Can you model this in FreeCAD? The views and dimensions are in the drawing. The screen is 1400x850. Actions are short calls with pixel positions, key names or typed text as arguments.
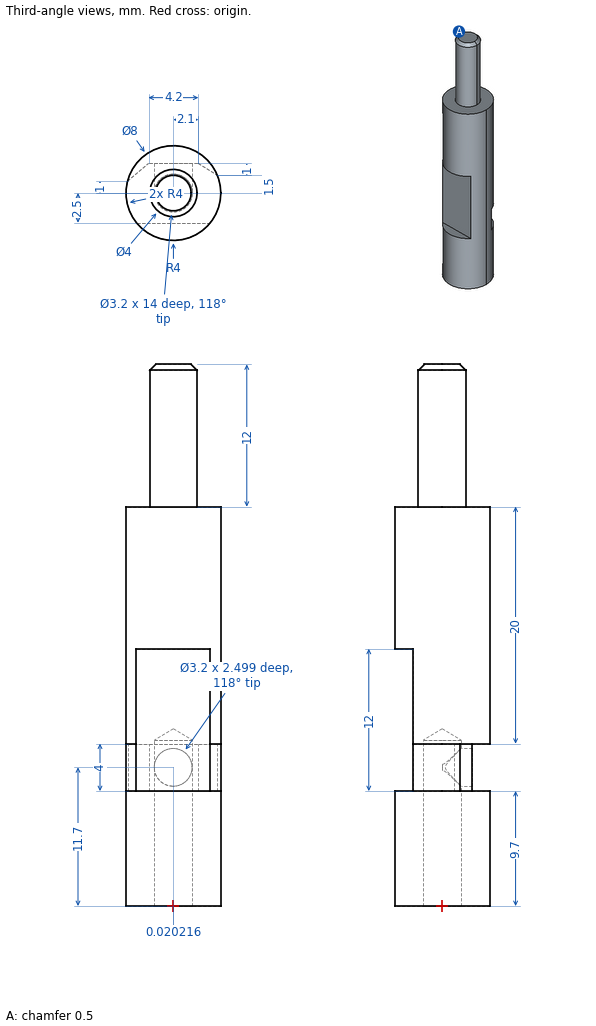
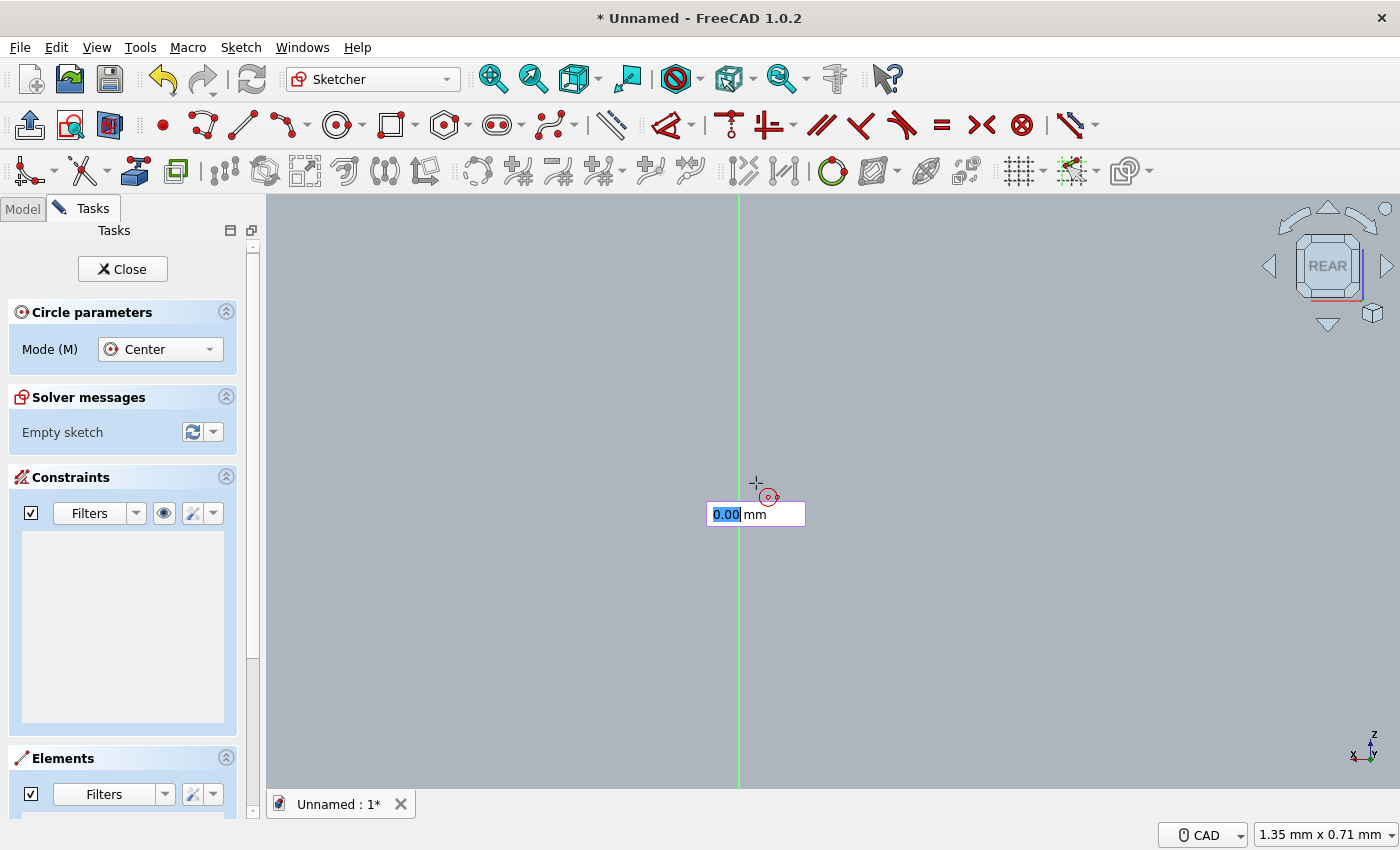
scroll(766, 493, down, 10)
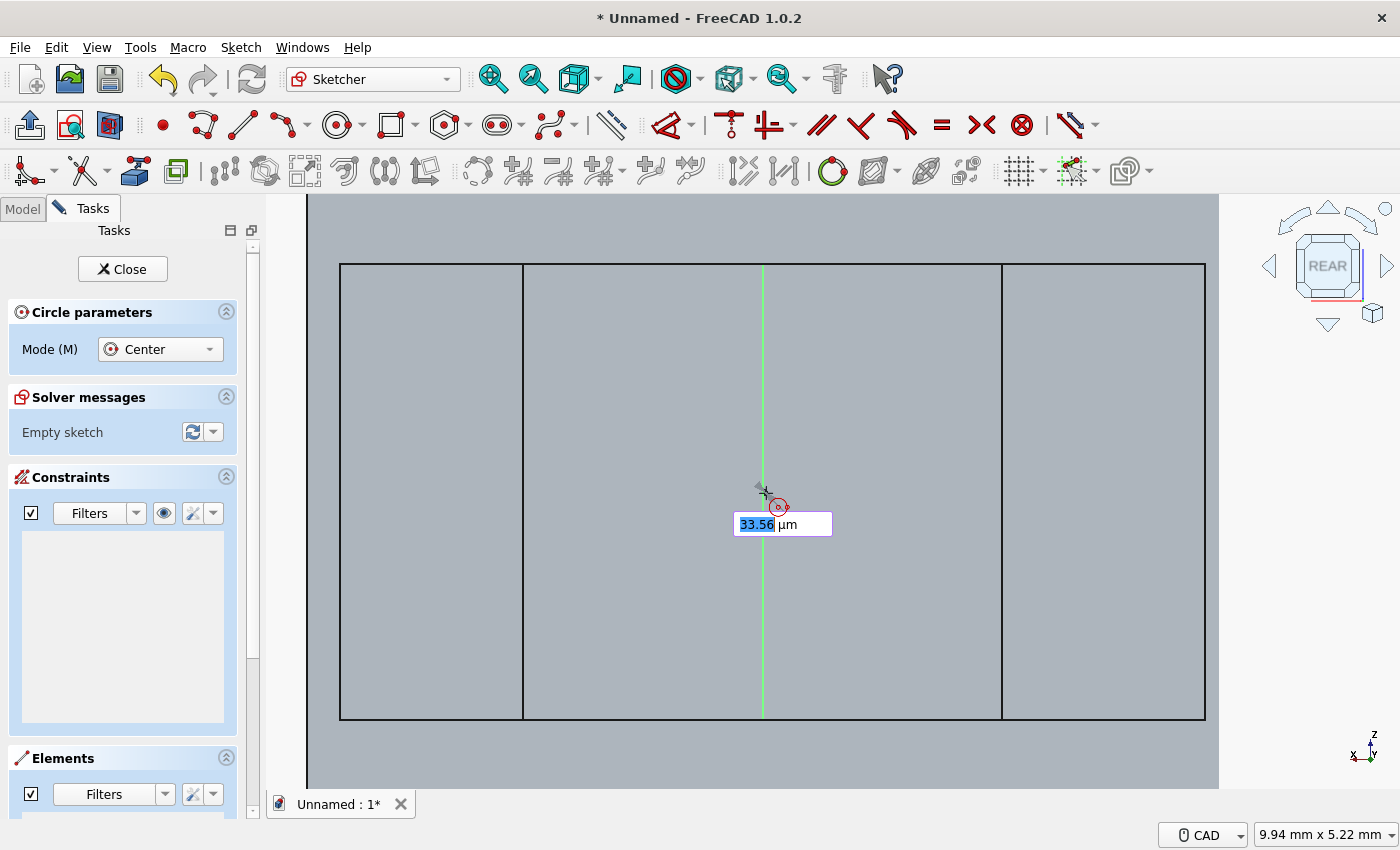
click(894, 363)
key(Escape)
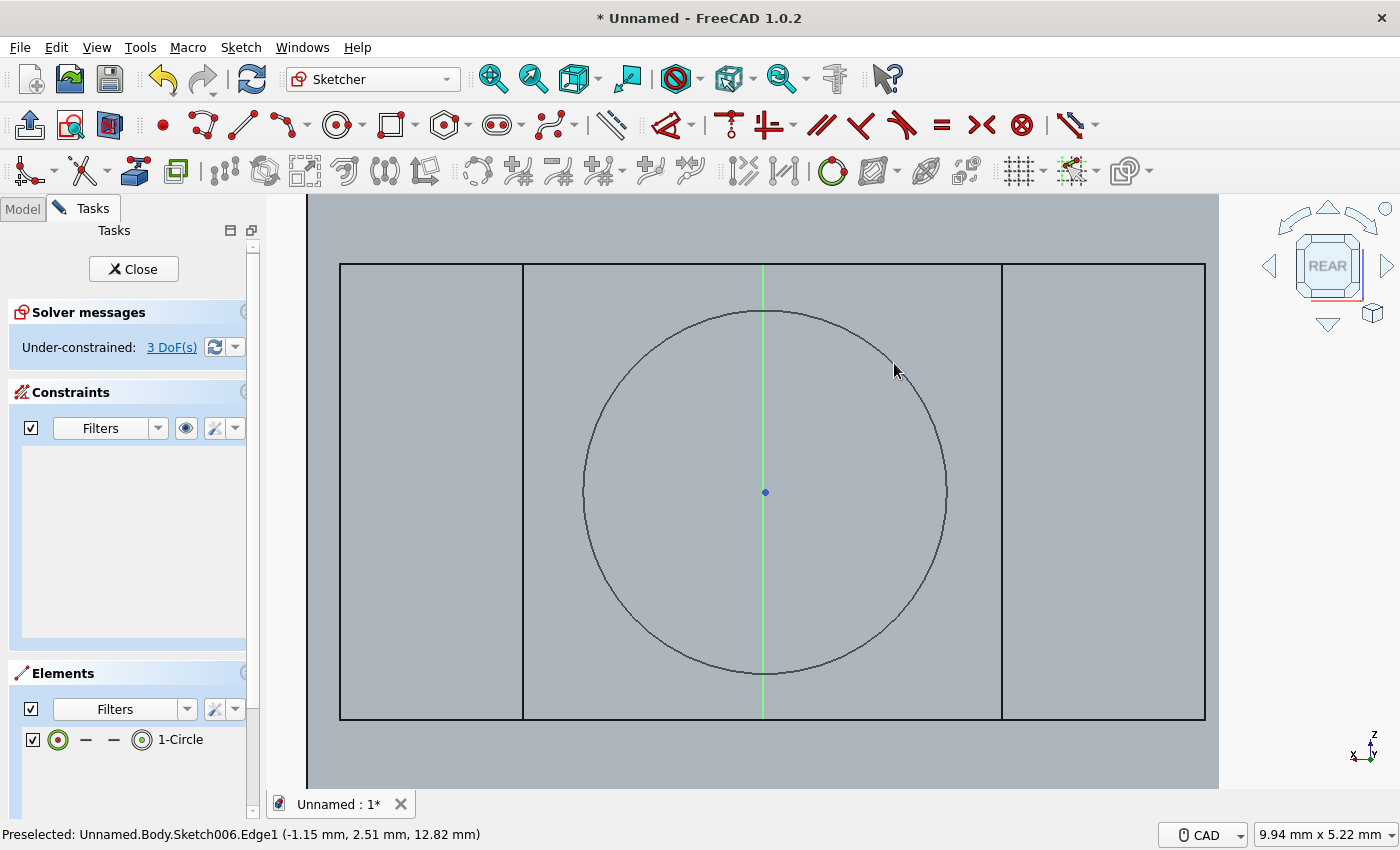
key(d)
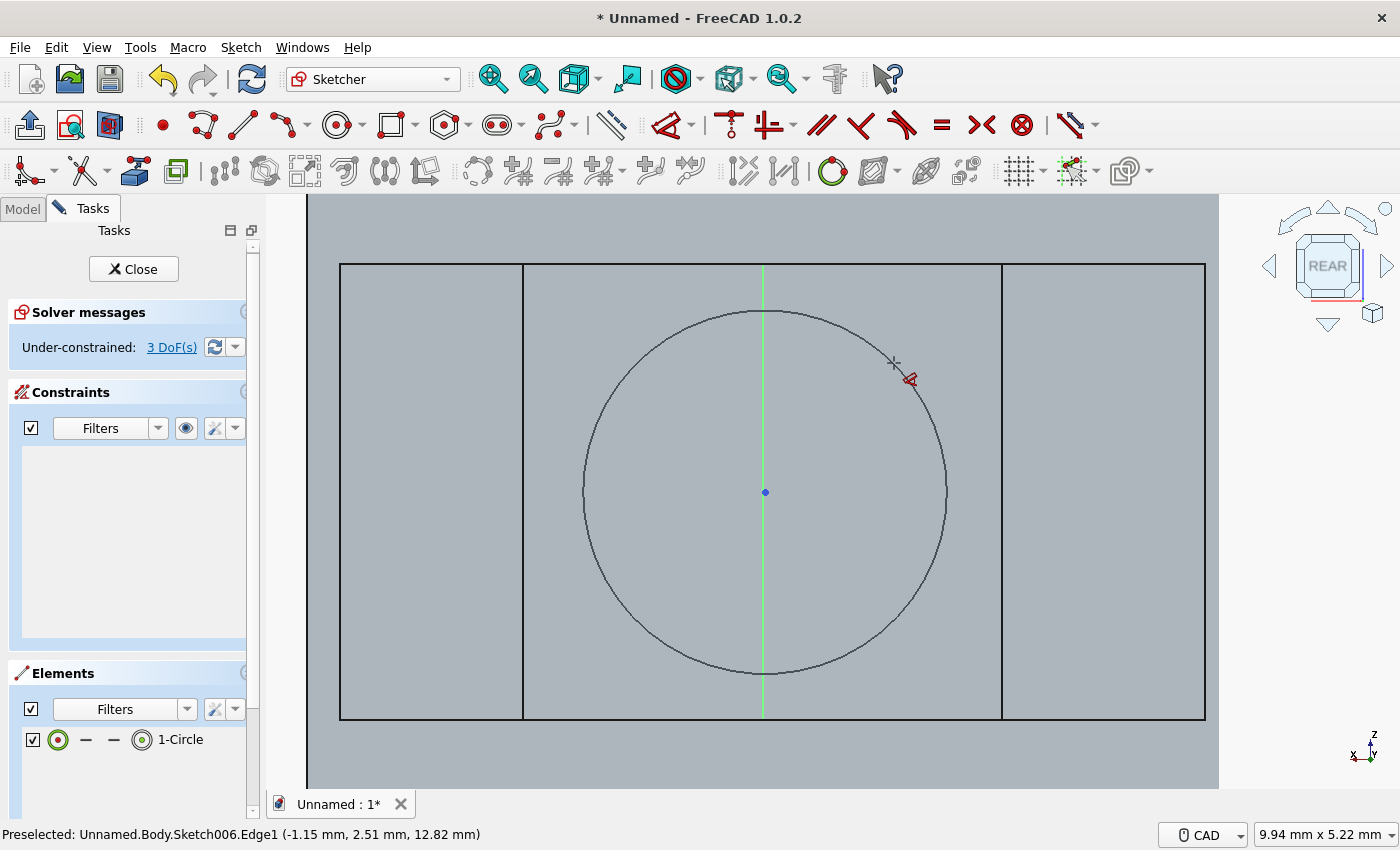
click(893, 363)
click(916, 340)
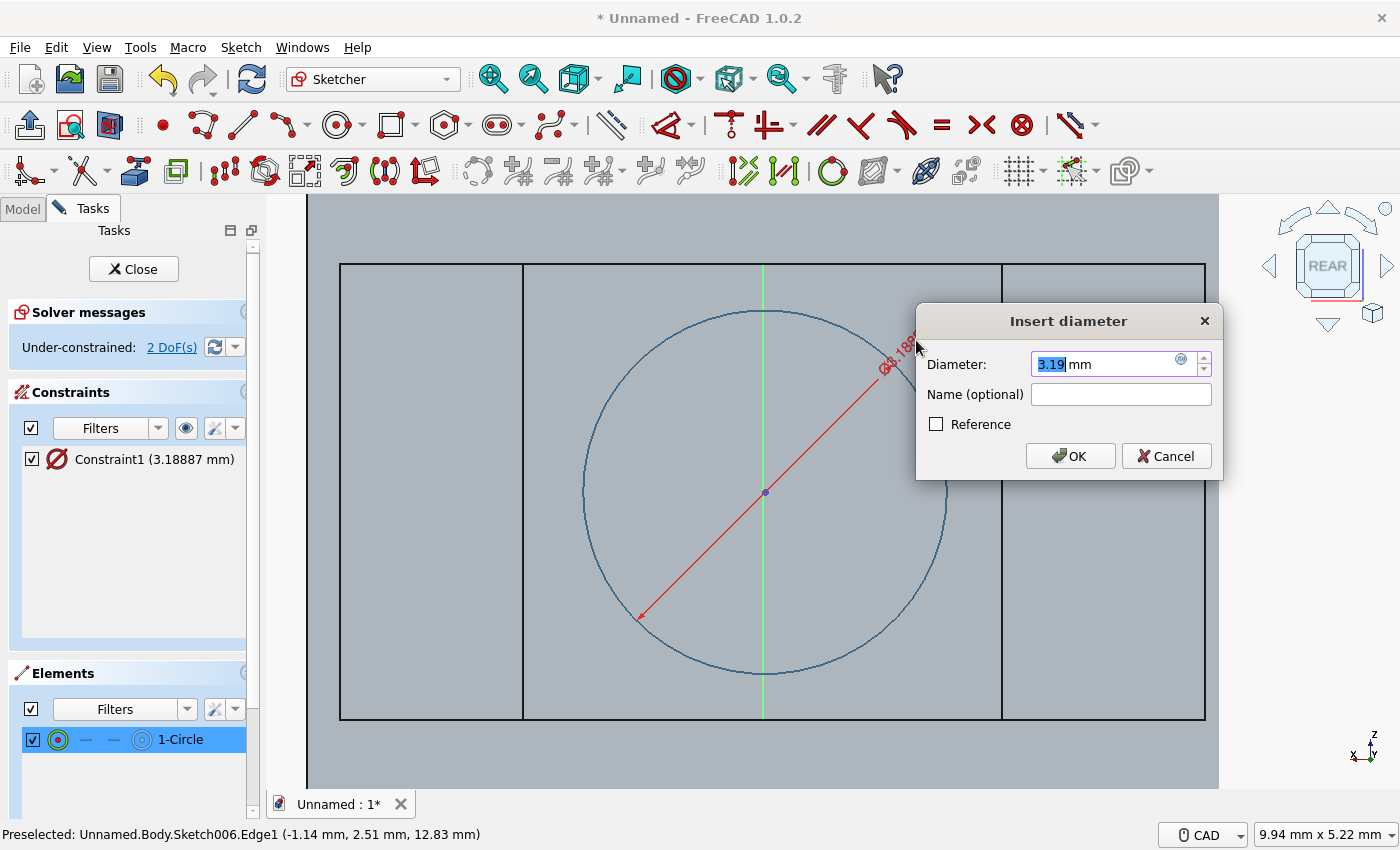
text(3.2)
key(Return)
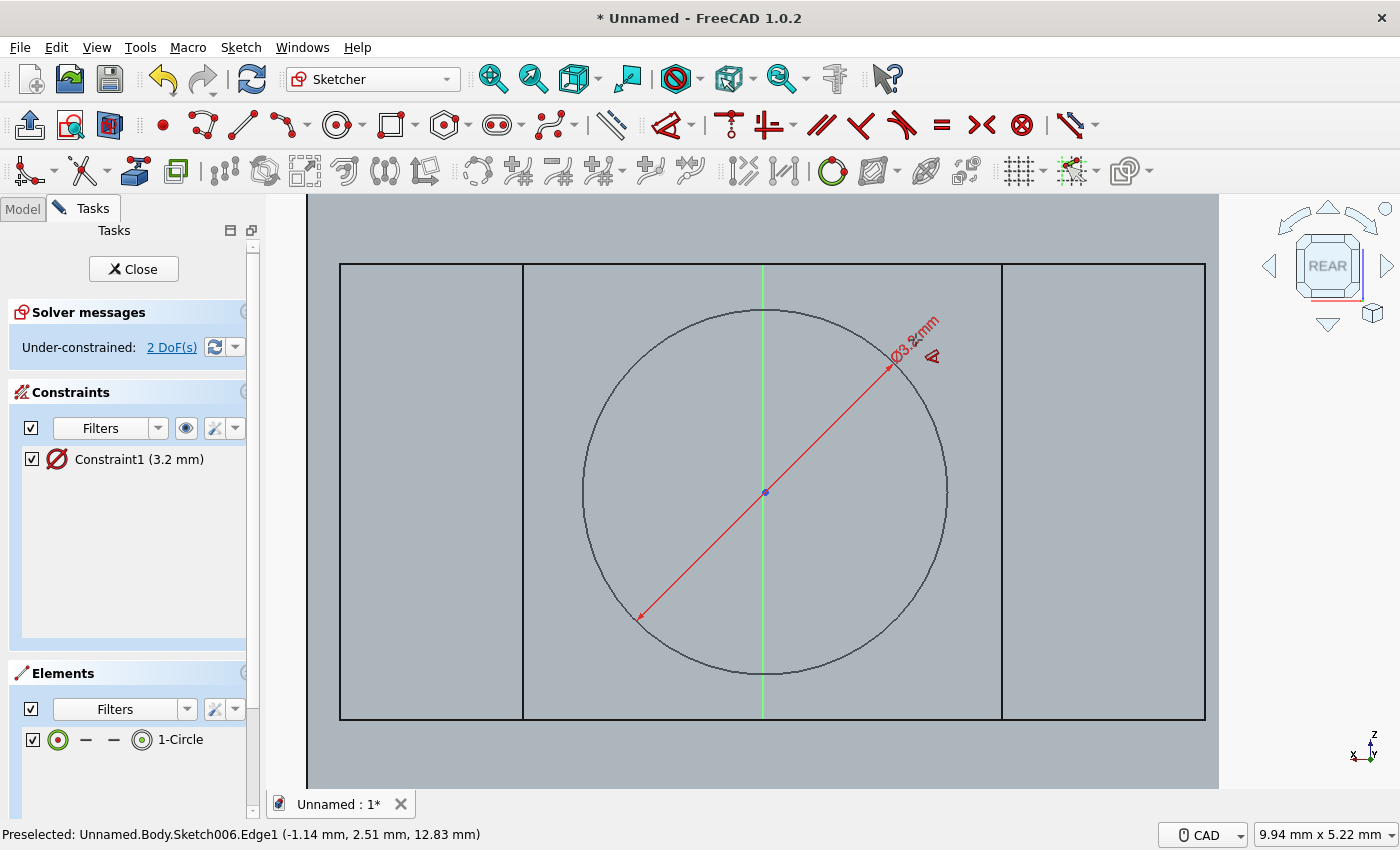
click(765, 492)
click(729, 627)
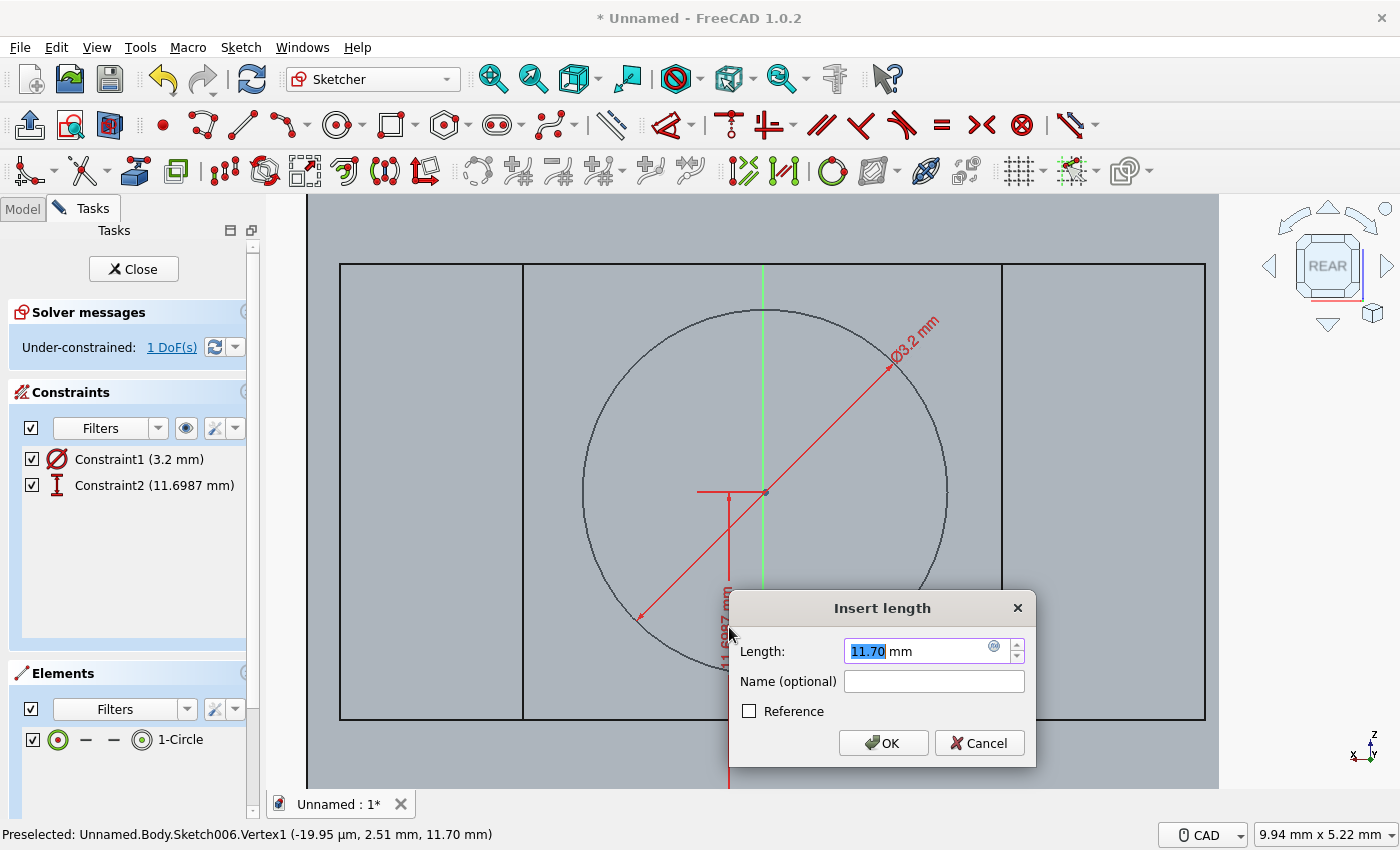
text(11.7)
key(Return)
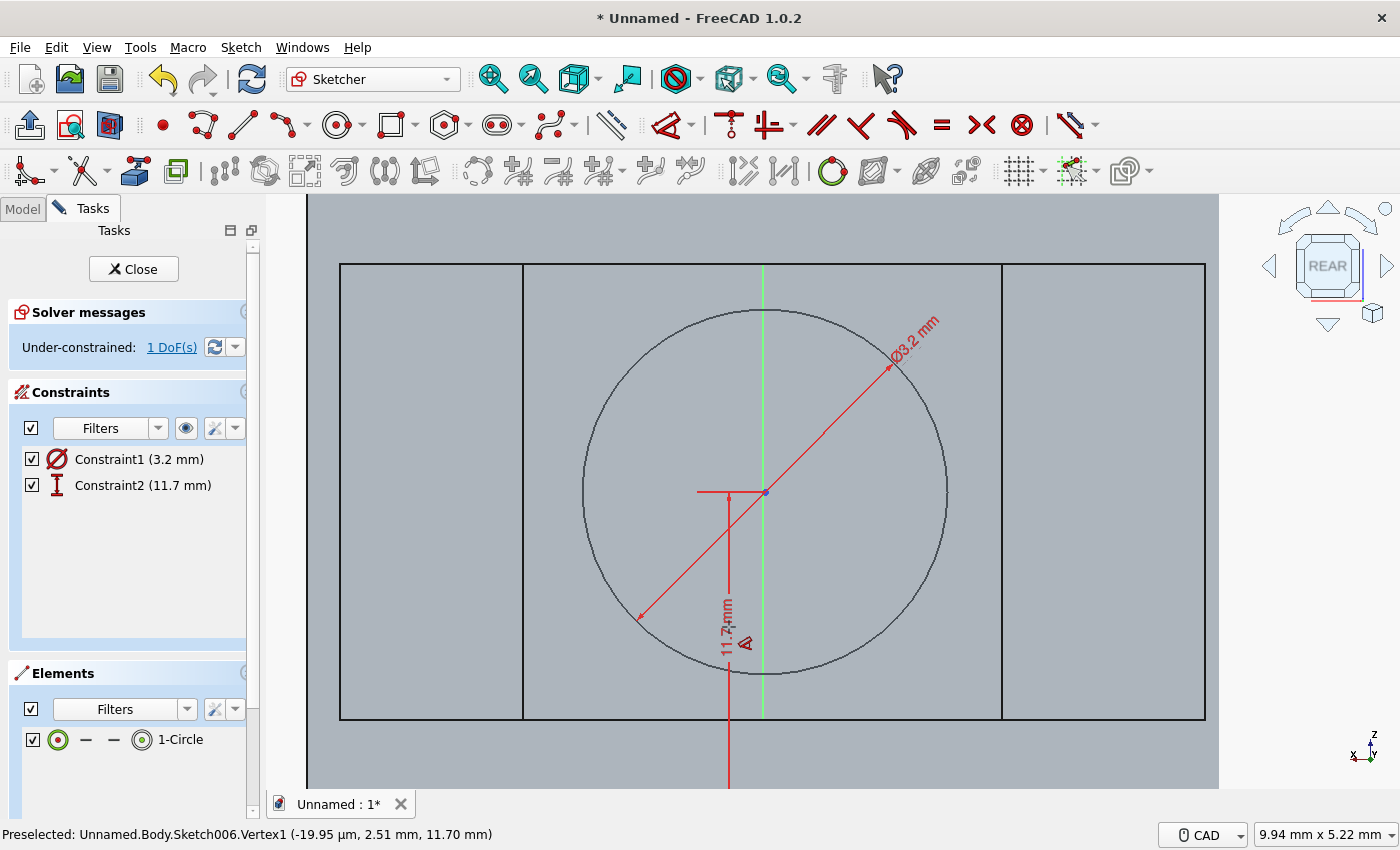
scroll(765, 492, up, 15)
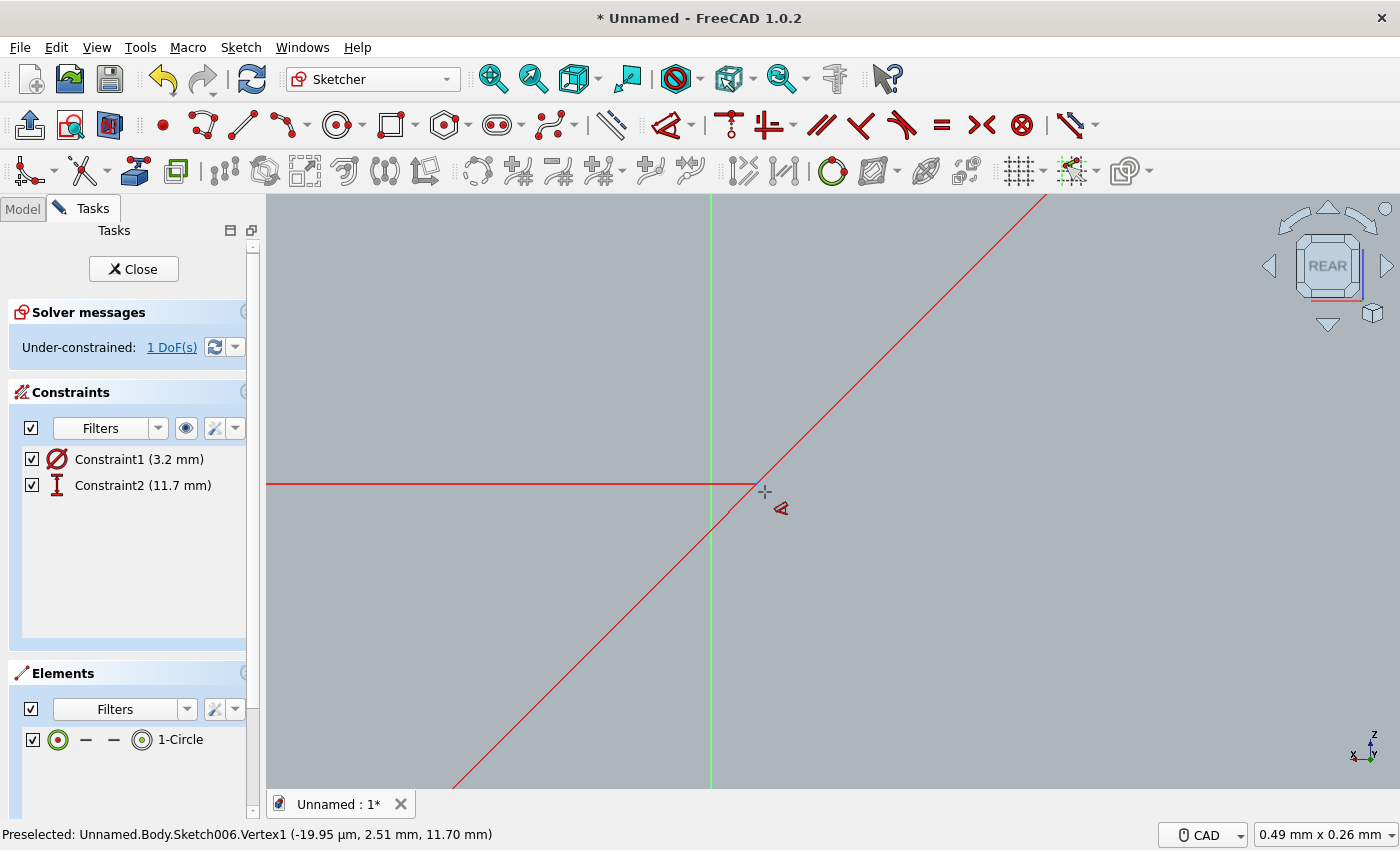
click(757, 484)
click(734, 450)